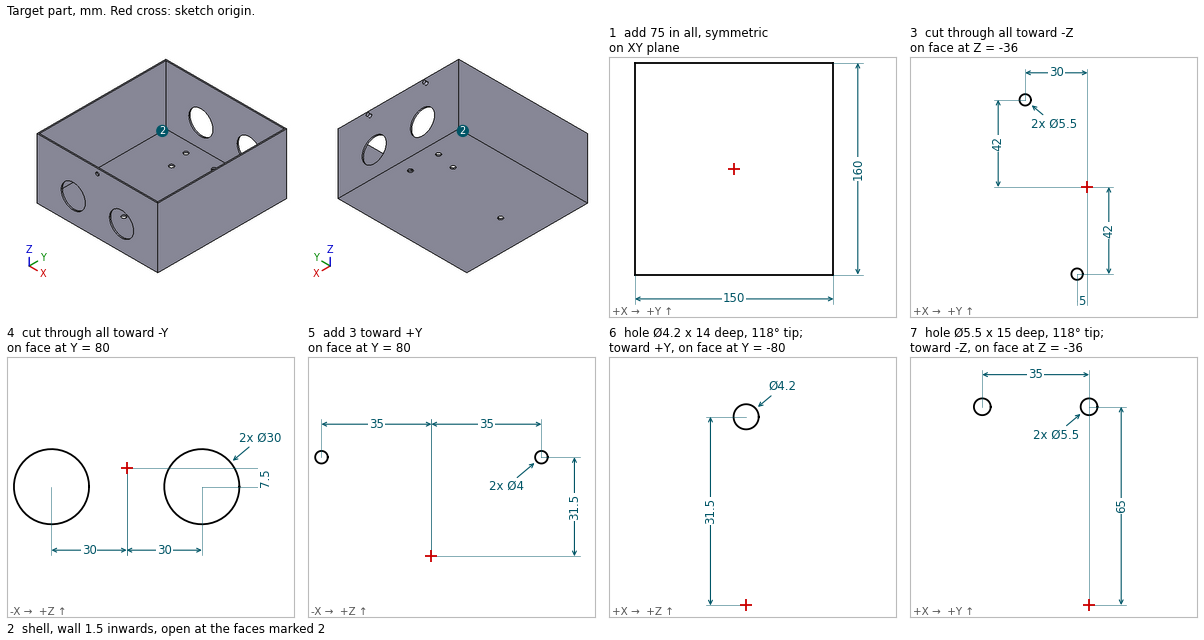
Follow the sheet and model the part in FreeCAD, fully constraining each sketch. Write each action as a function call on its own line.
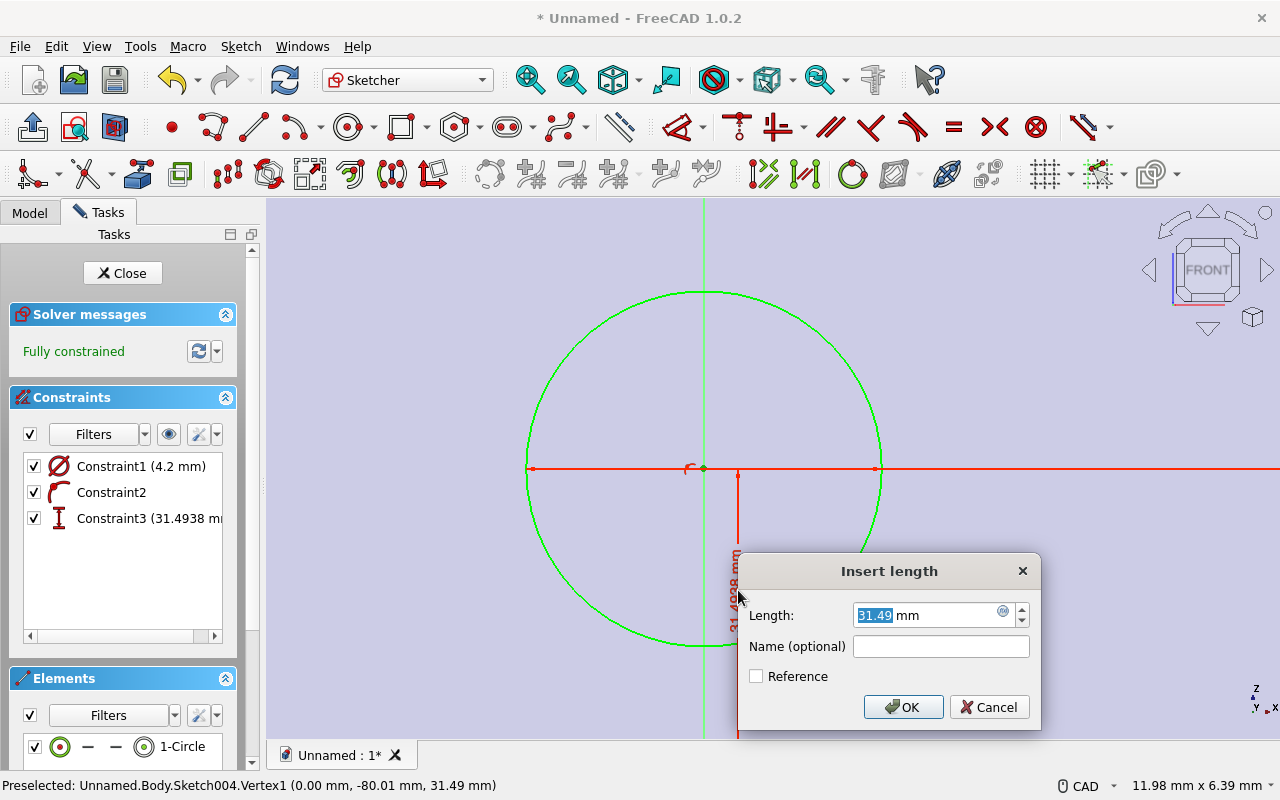
text(31.5)
key(Return)
key(Escape)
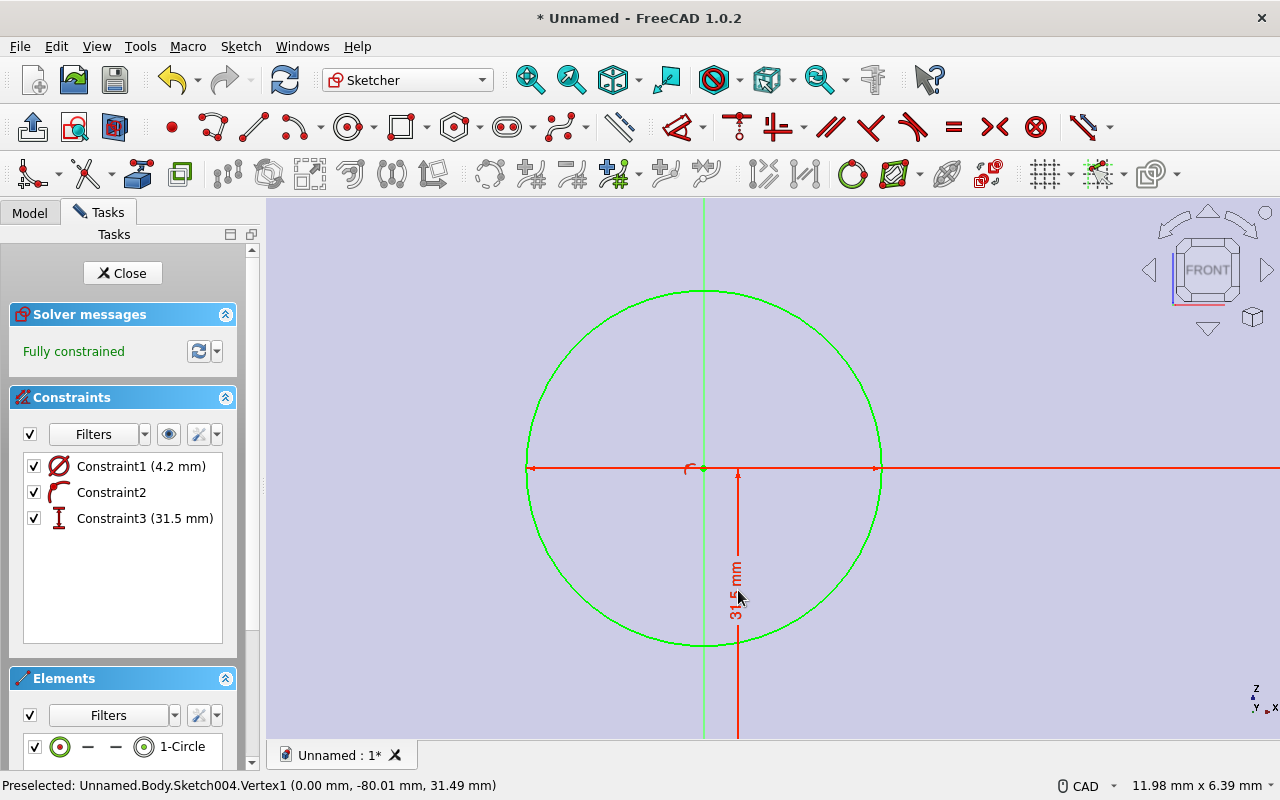
click(123, 273)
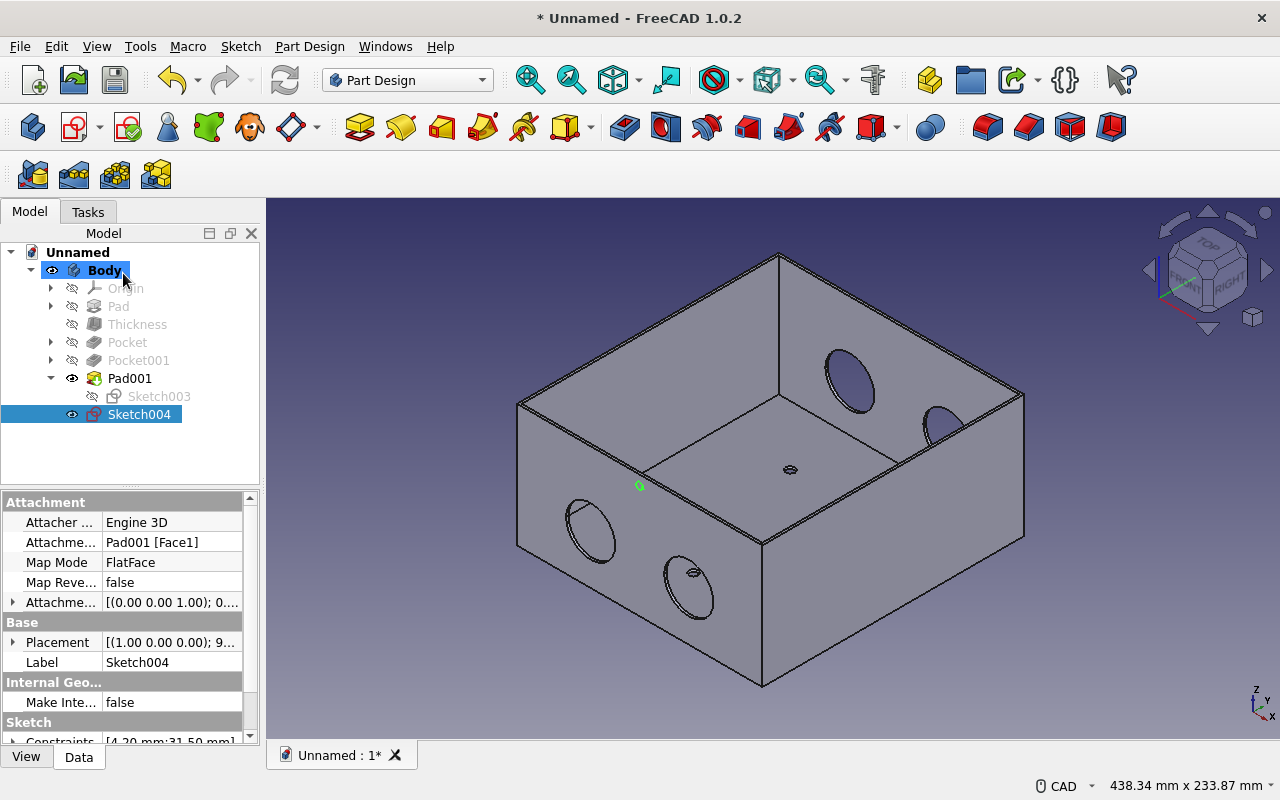
click(666, 128)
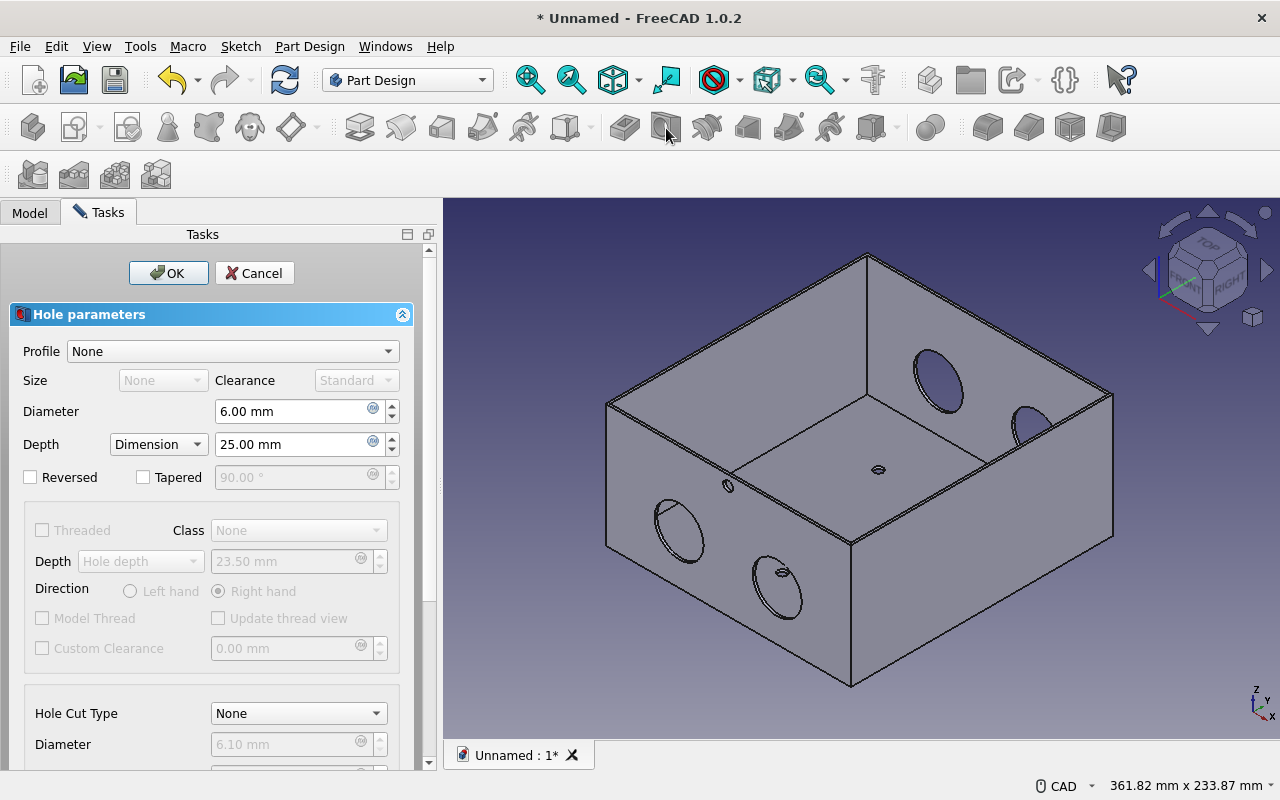
triple_click(300, 412)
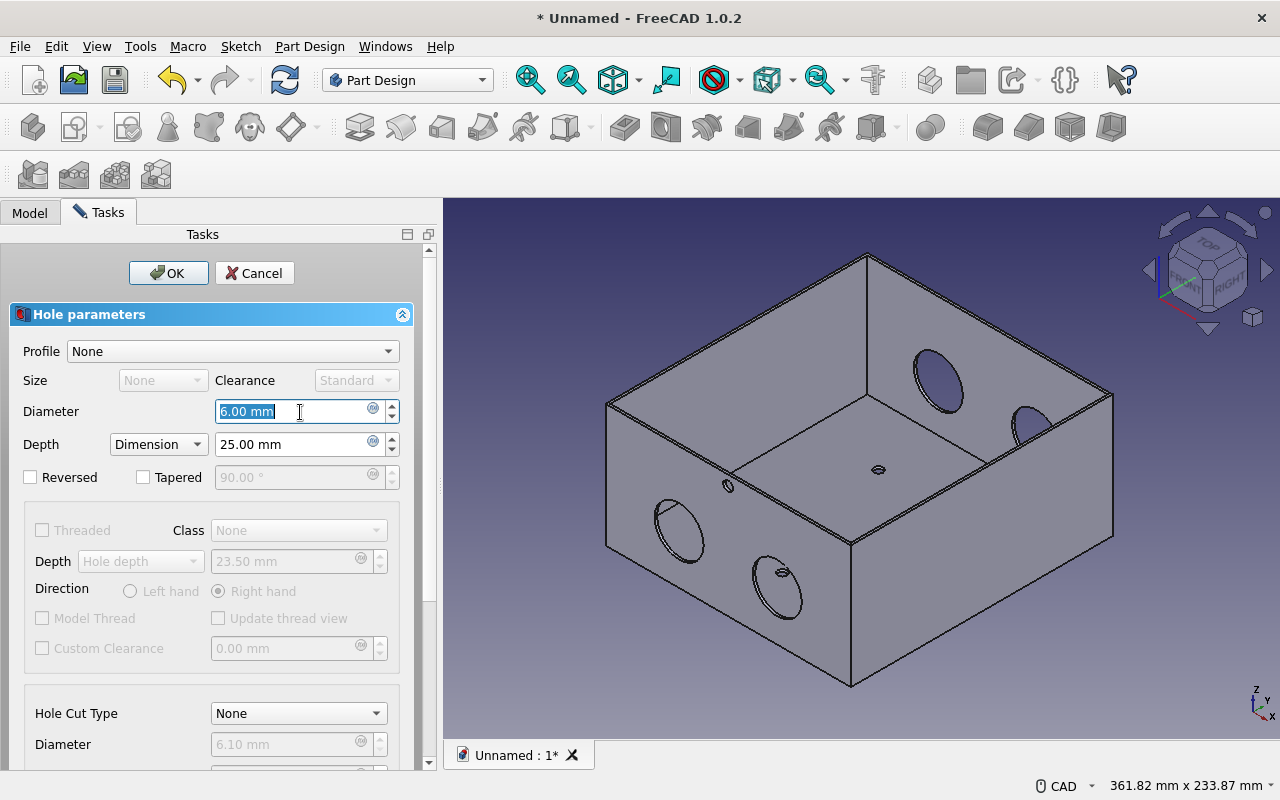
text(4.2)
key(Tab)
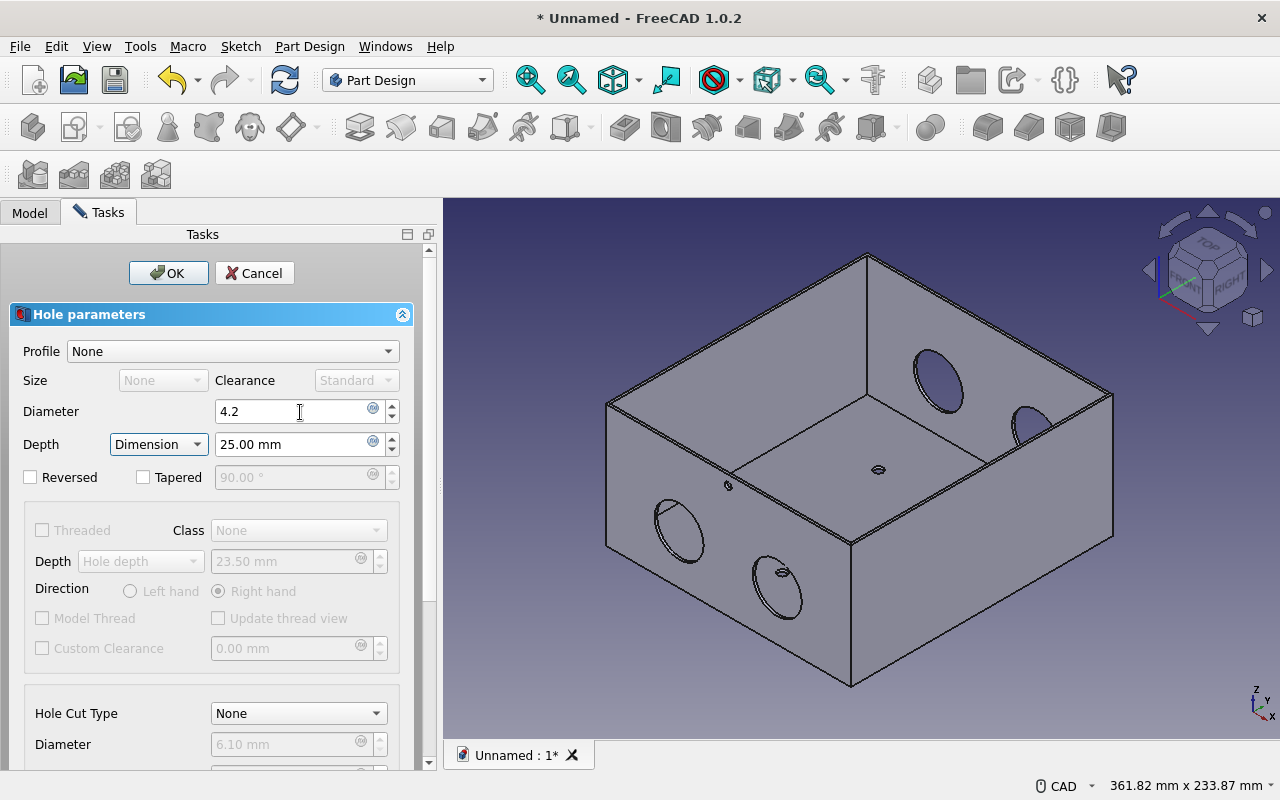
triple_click(300, 444)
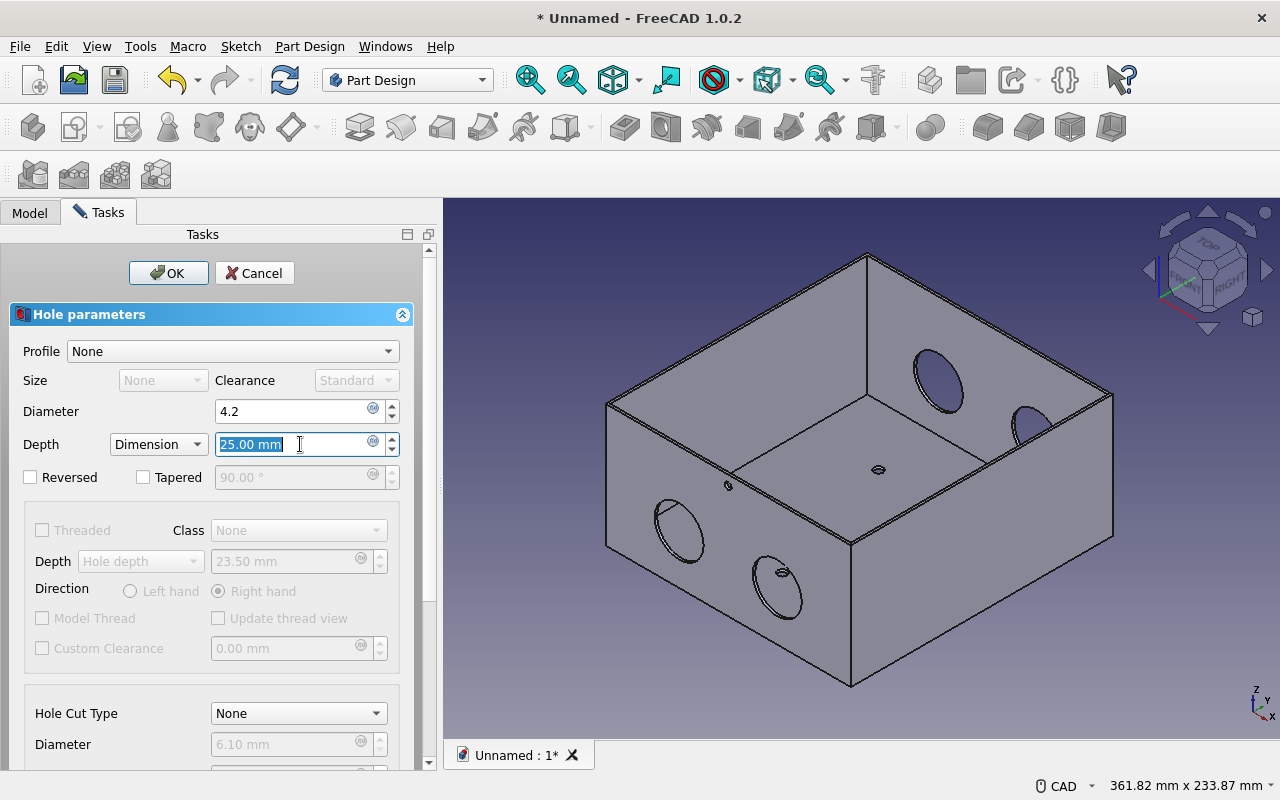
text(14)
key(Tab)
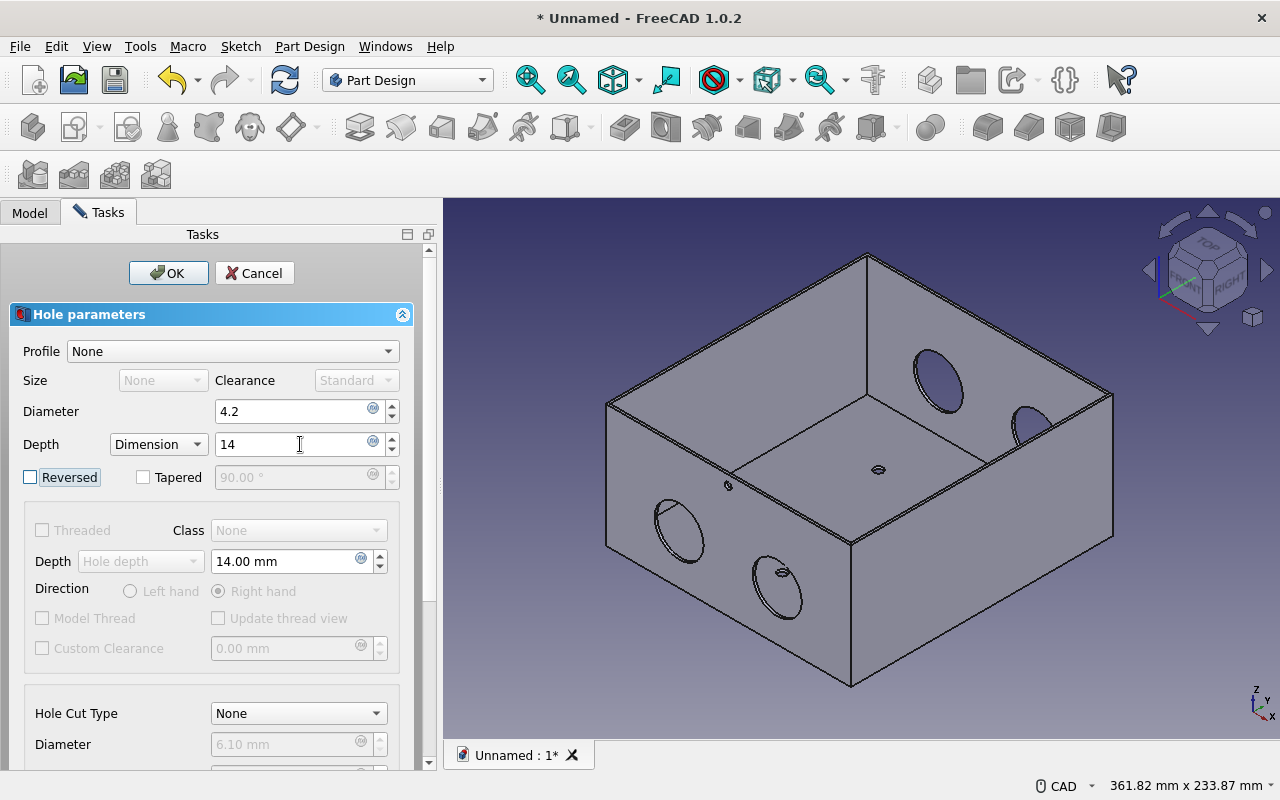
click(169, 273)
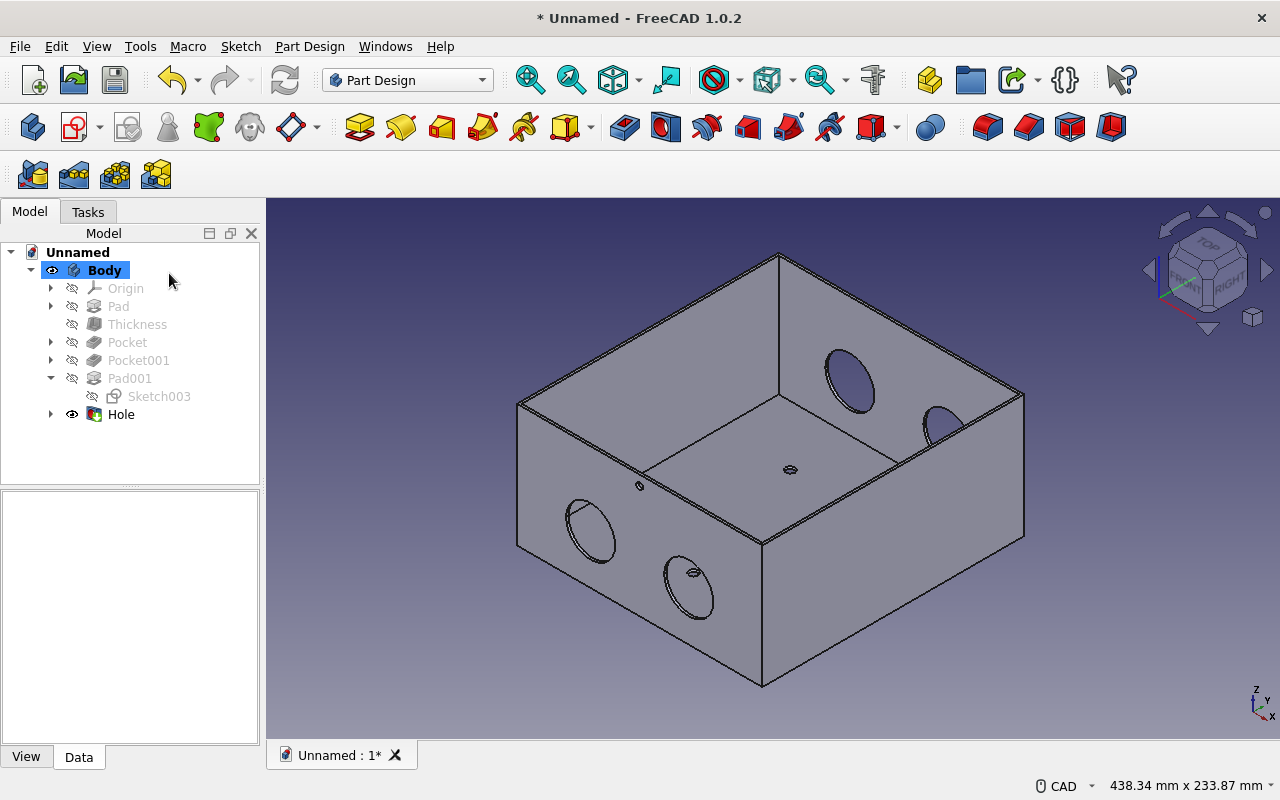
key(2)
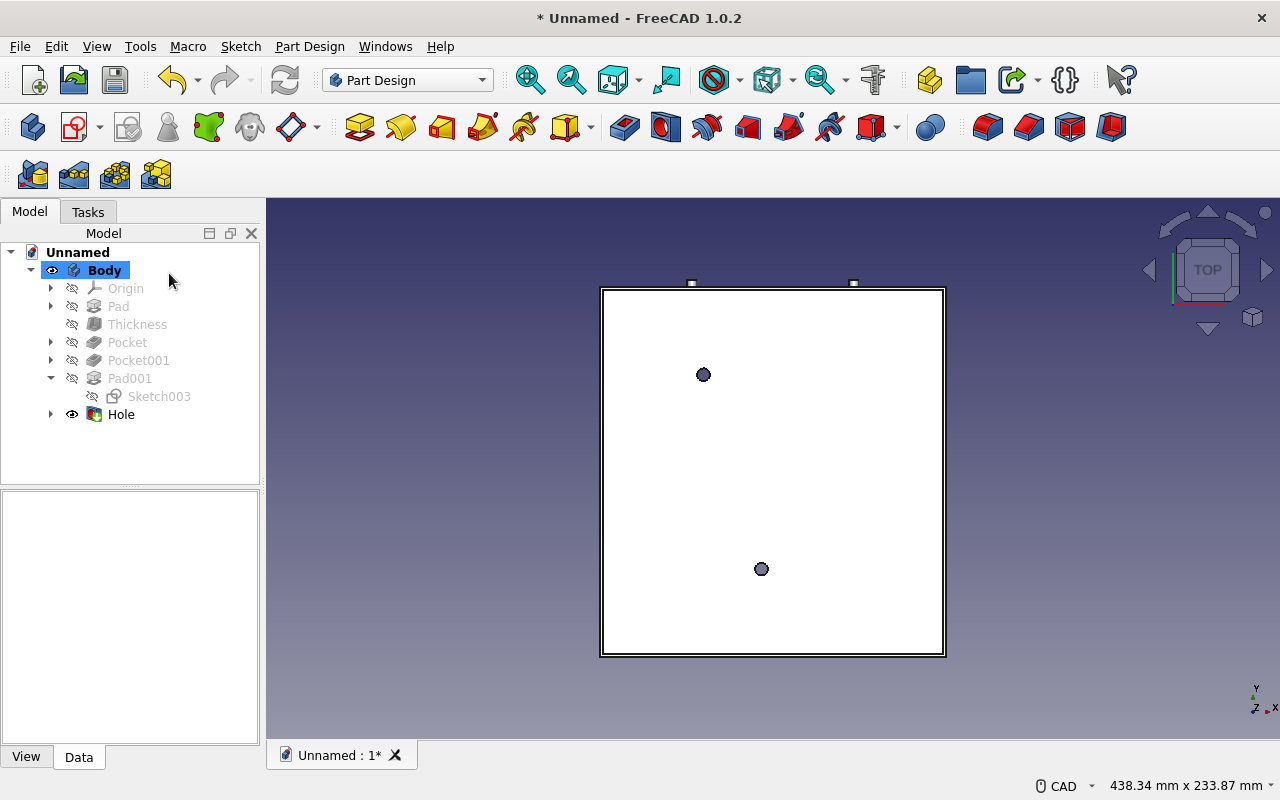
click(822, 419)